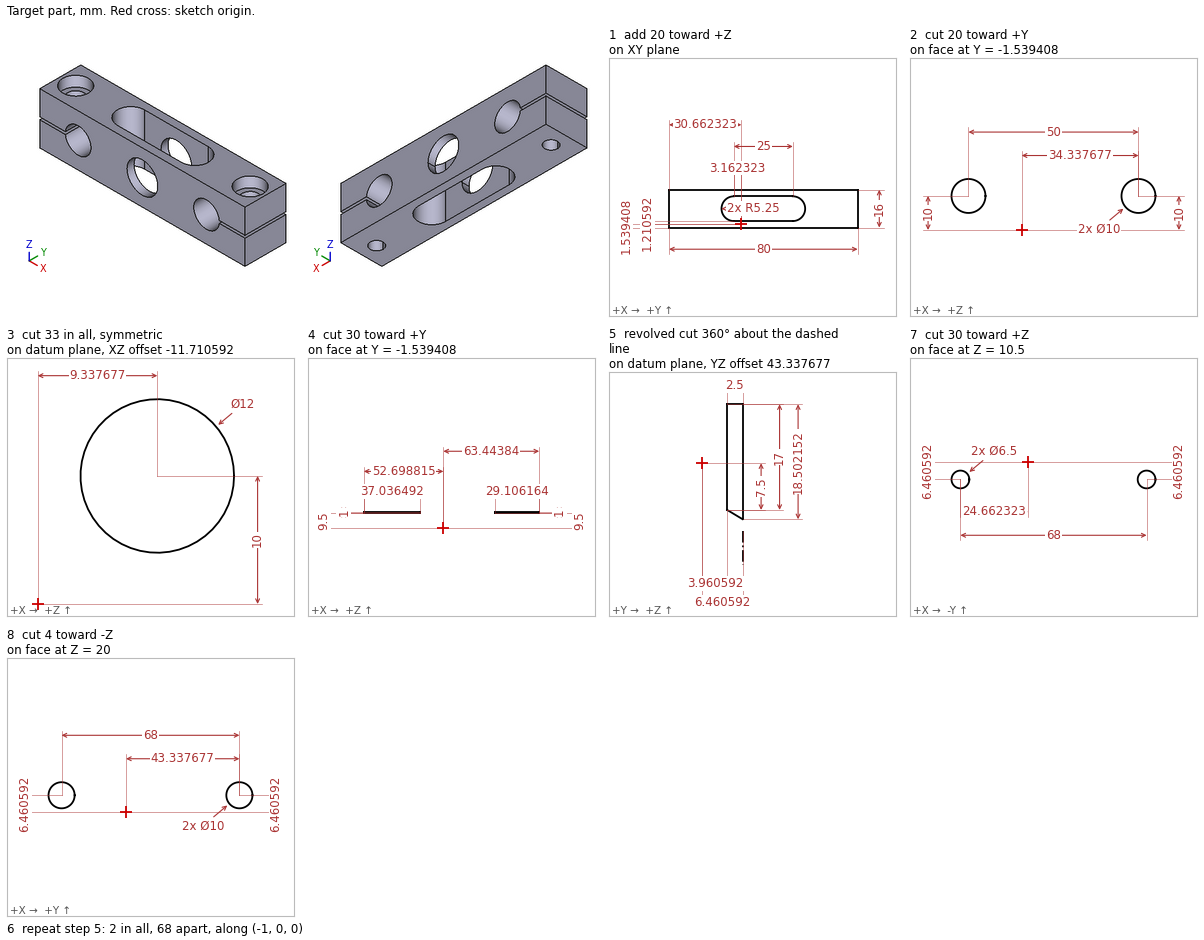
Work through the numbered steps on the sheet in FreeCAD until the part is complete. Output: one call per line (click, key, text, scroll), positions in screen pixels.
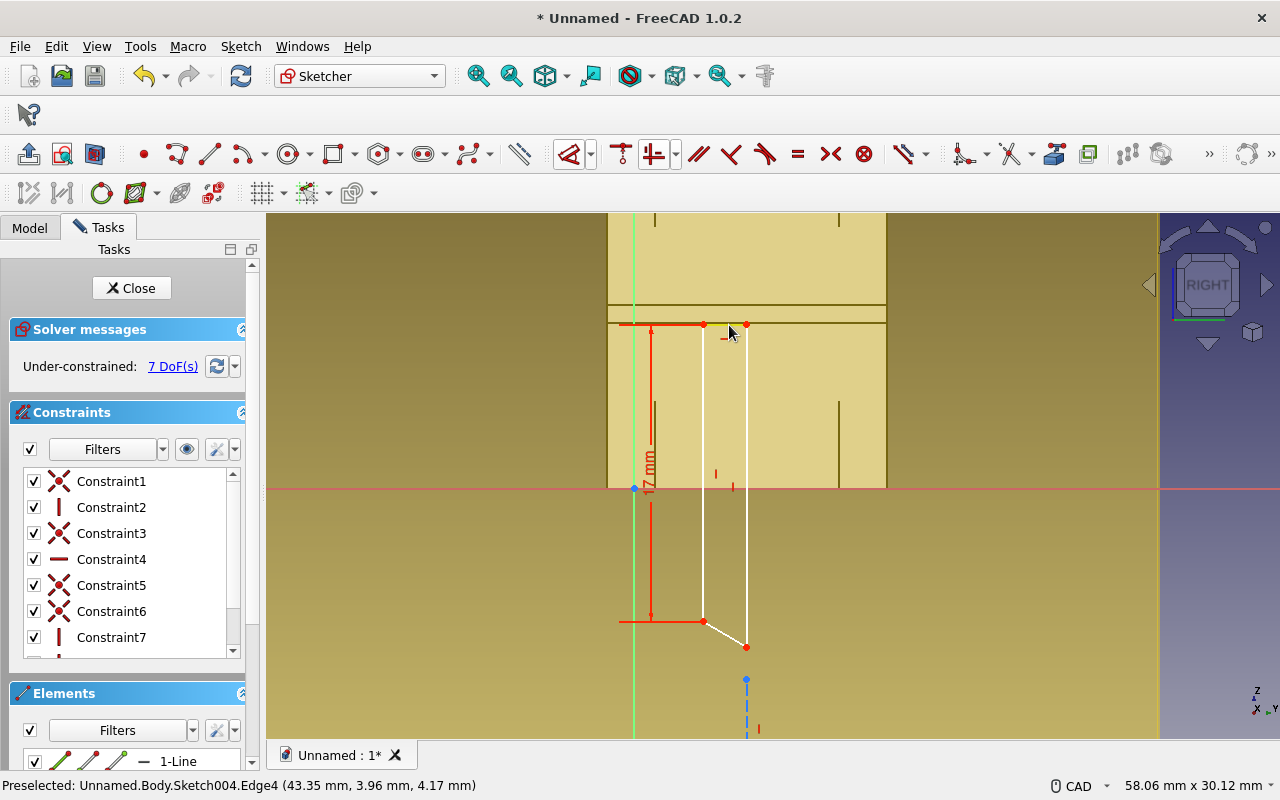
click(729, 325)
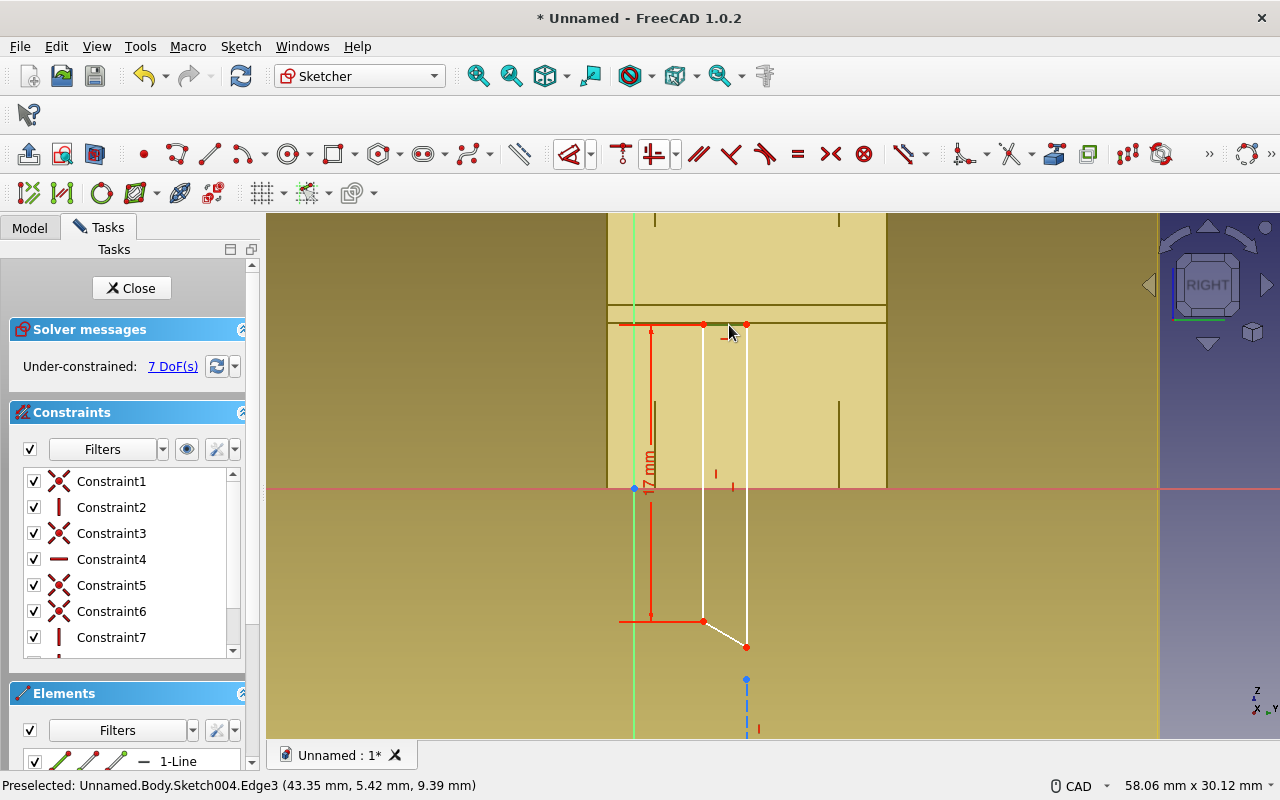
key(l)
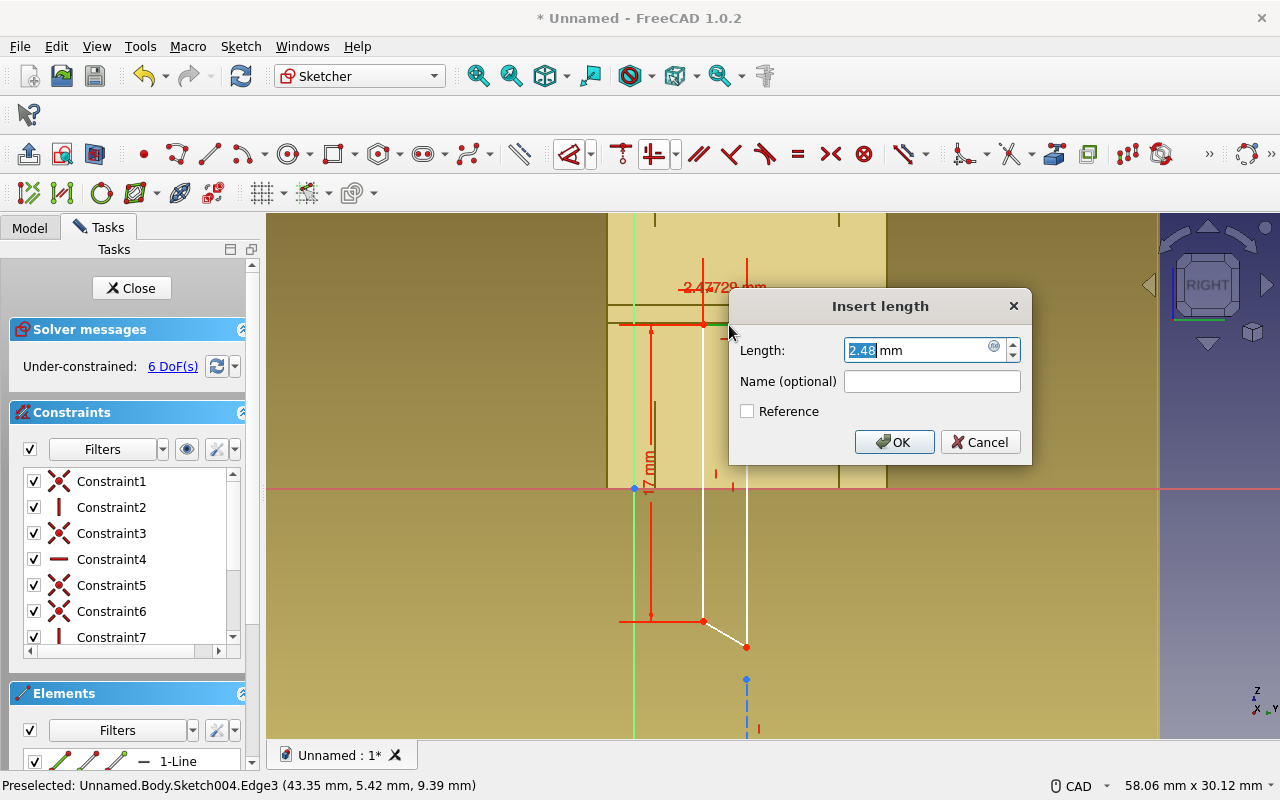
text(2.5)
key(Return)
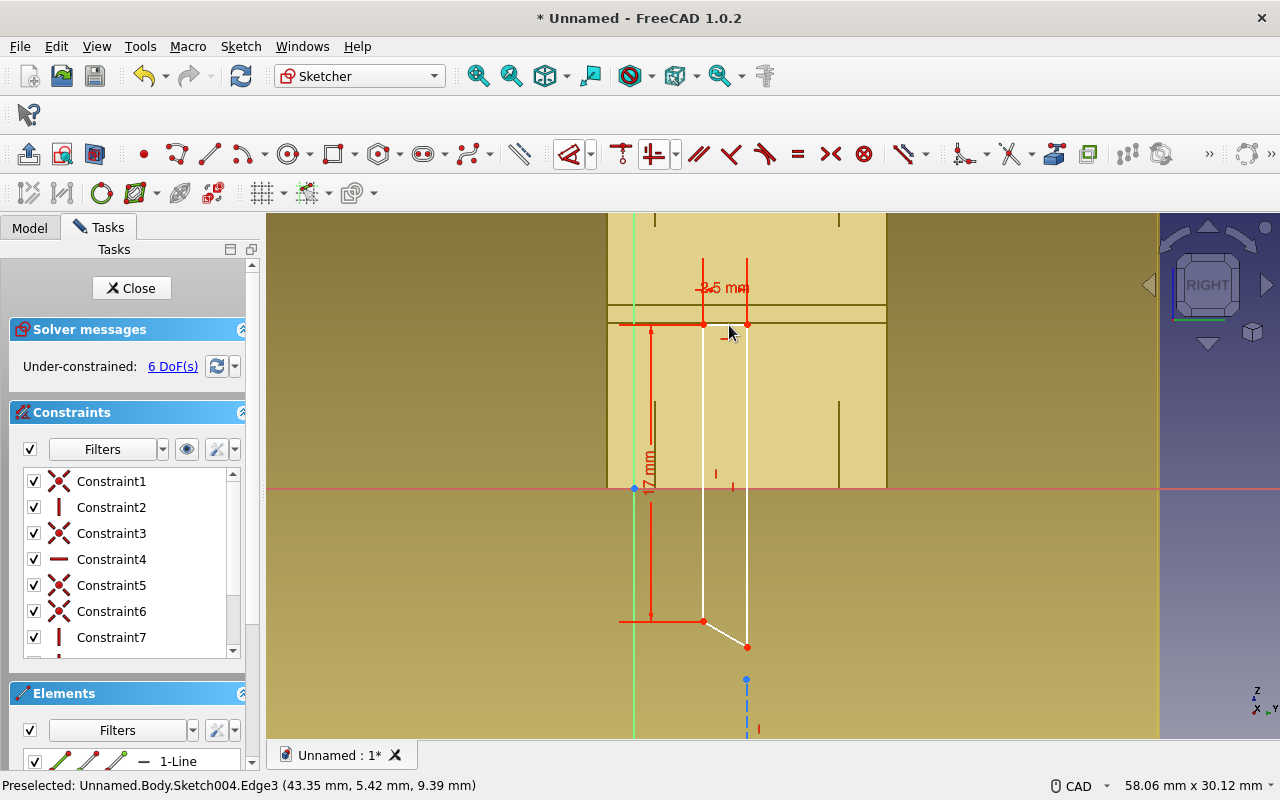
click(703, 622)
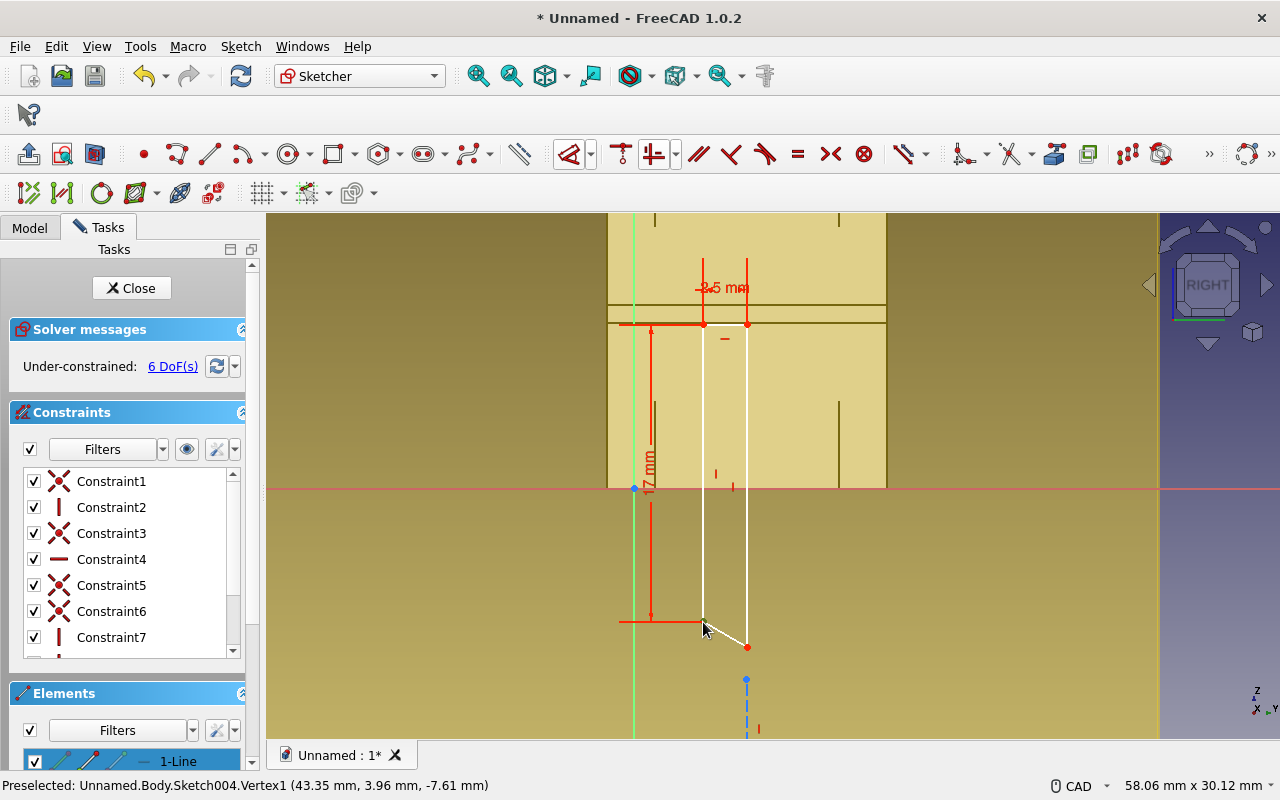
click(590, 154)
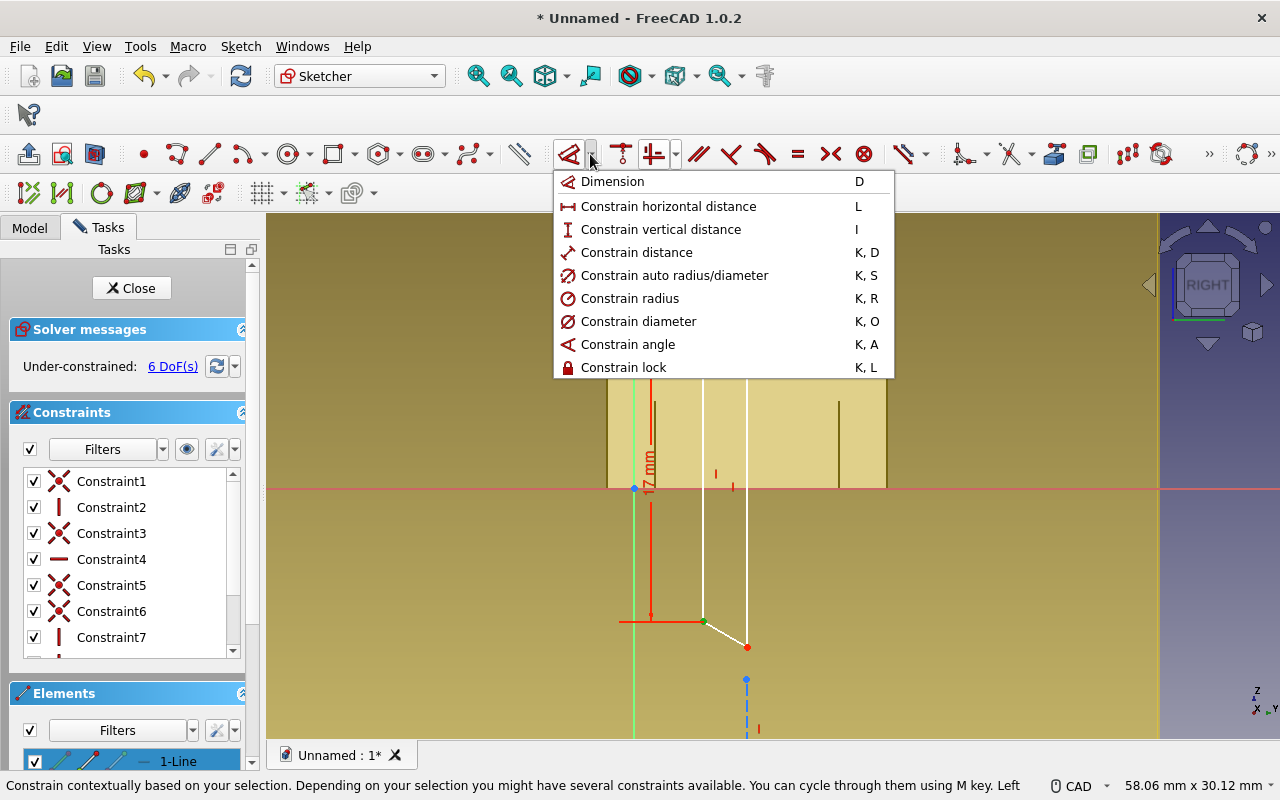
click(724, 230)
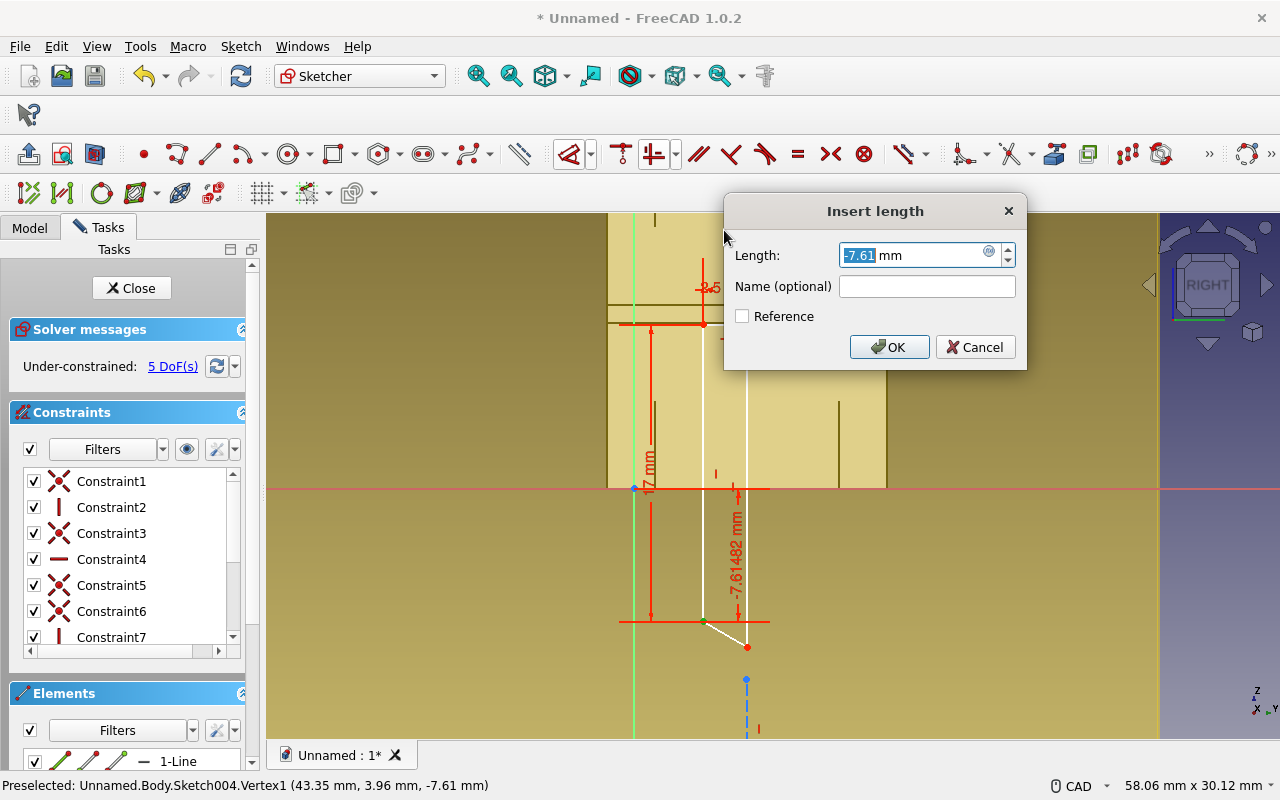
text(-7.5)
key(Return)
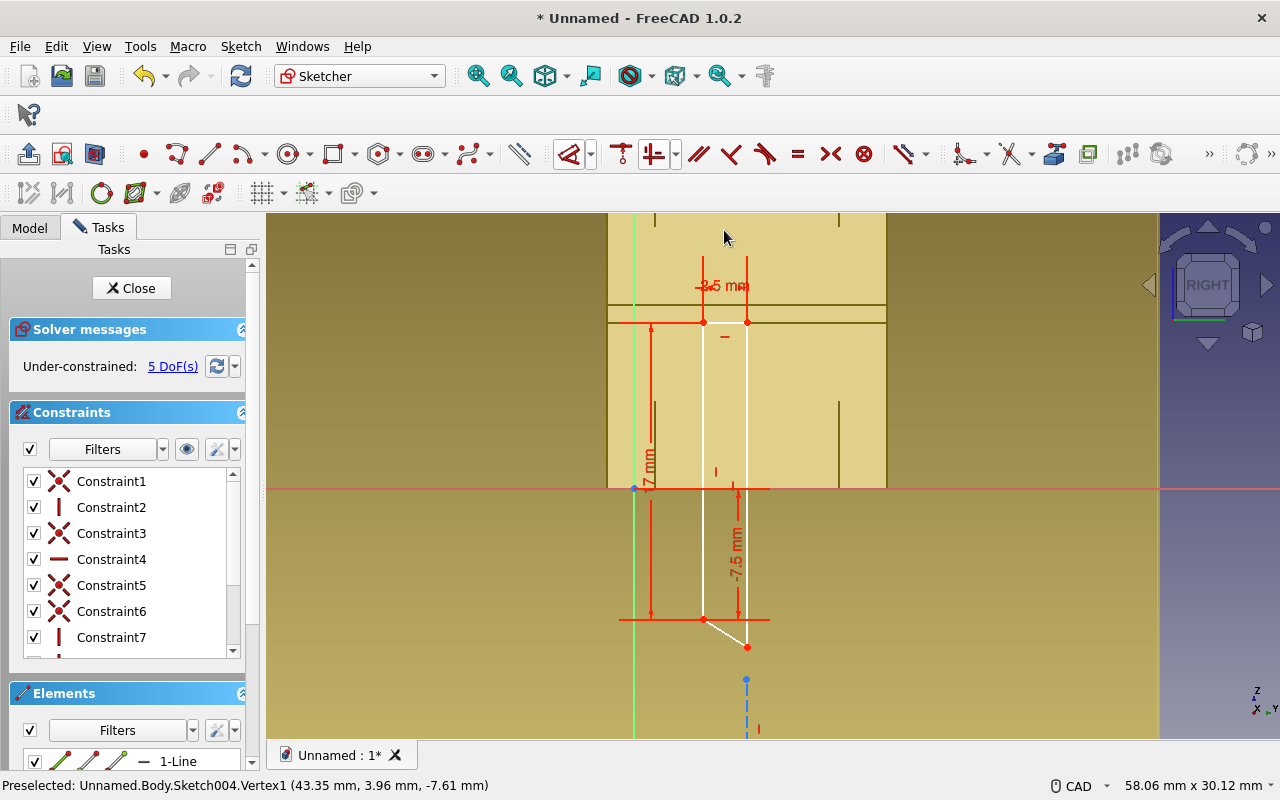
click(747, 550)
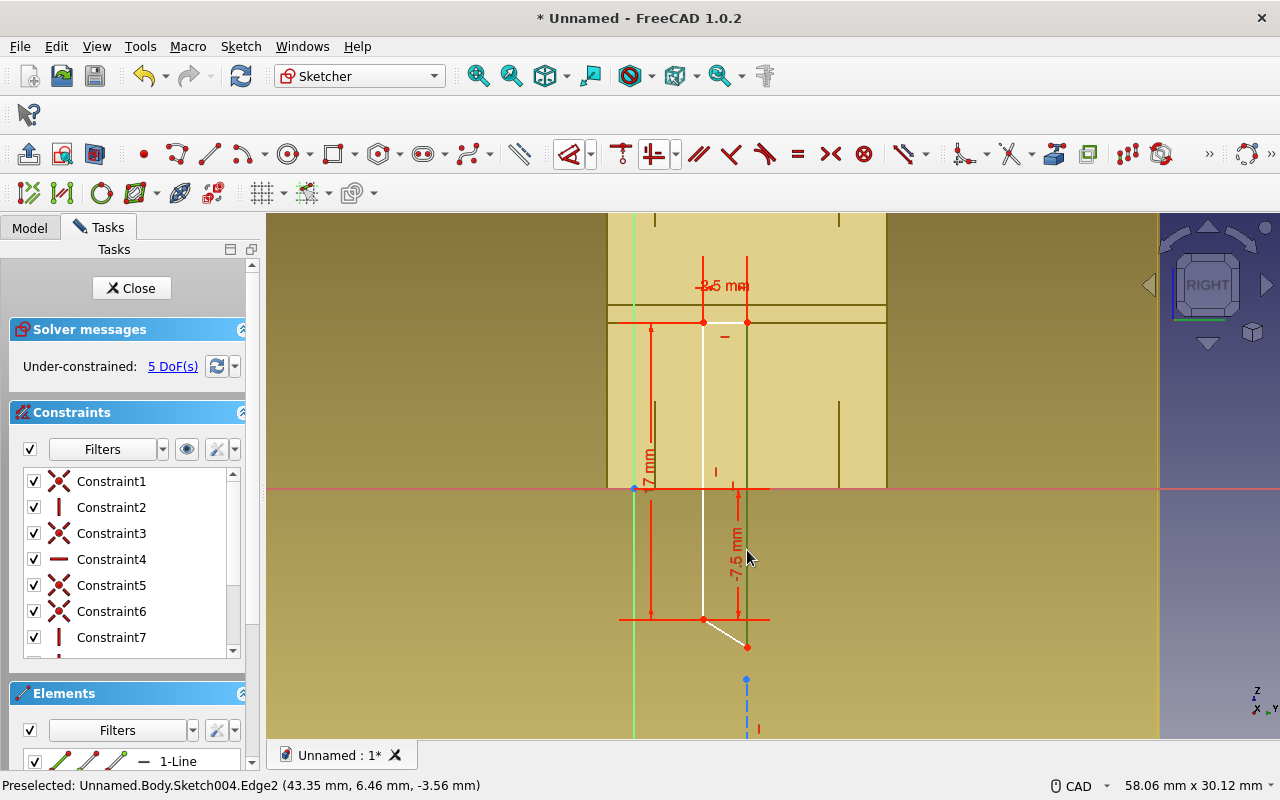
key(i)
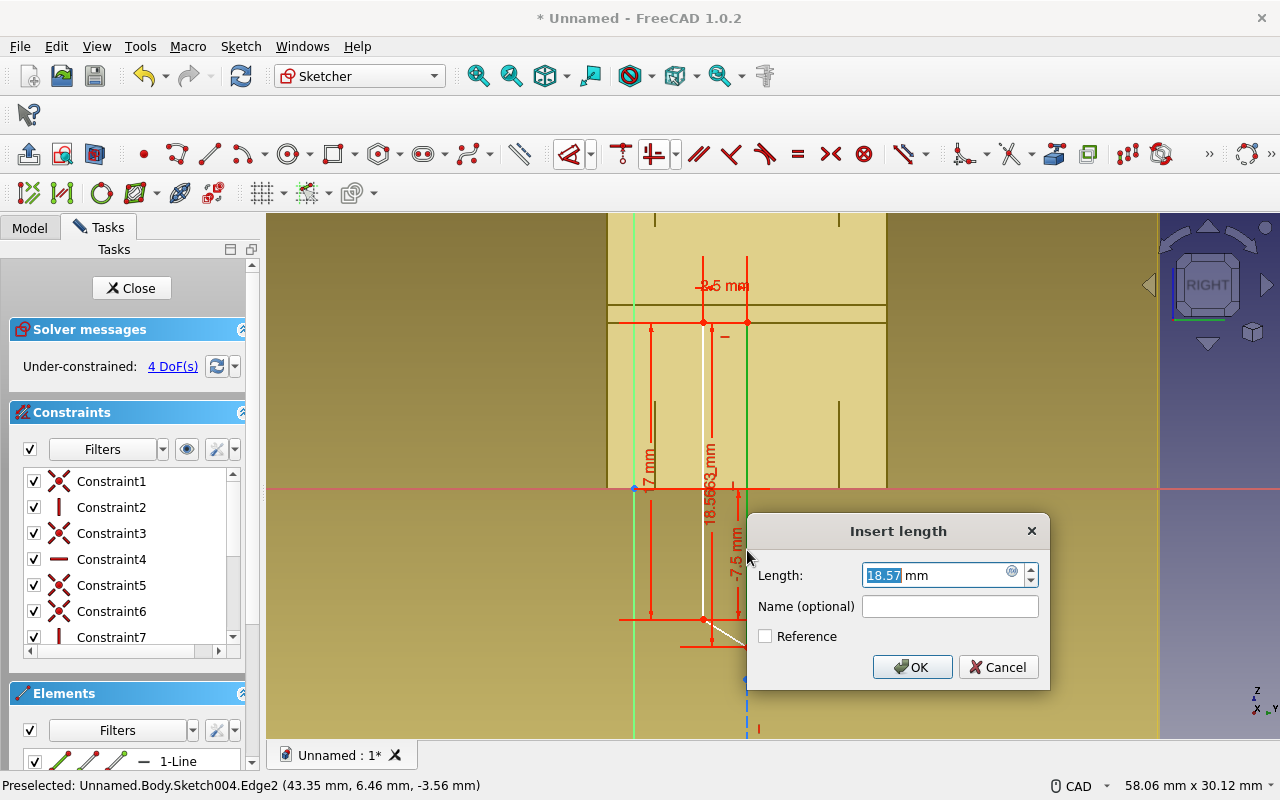
text(18.502152)
key(Return)